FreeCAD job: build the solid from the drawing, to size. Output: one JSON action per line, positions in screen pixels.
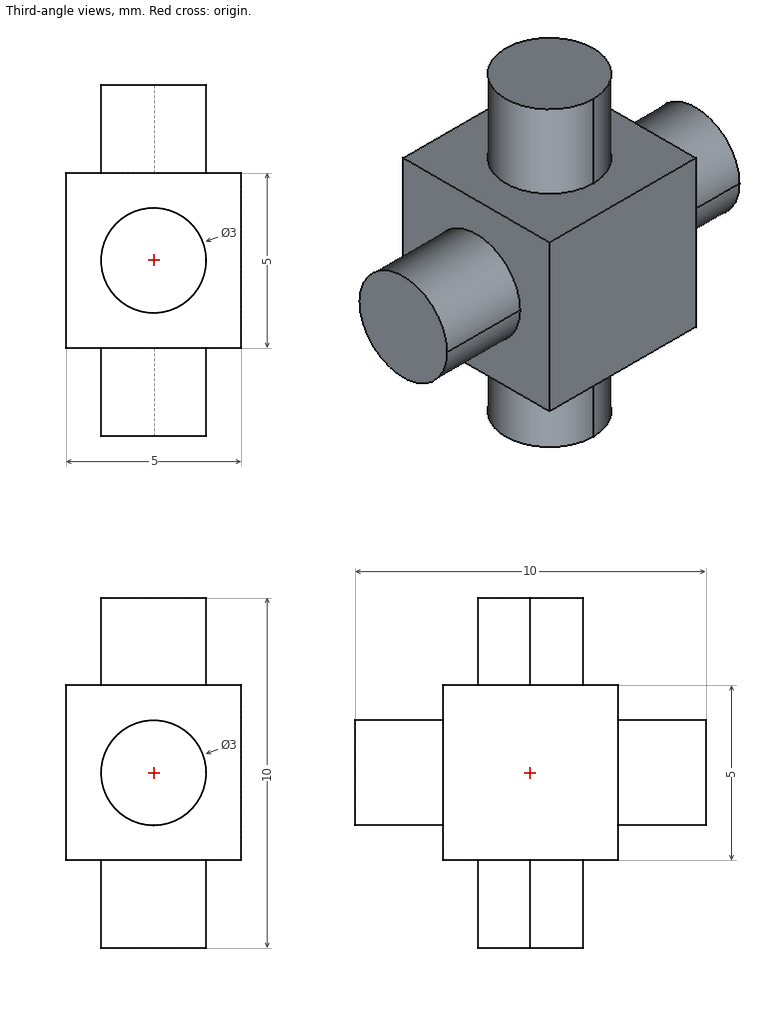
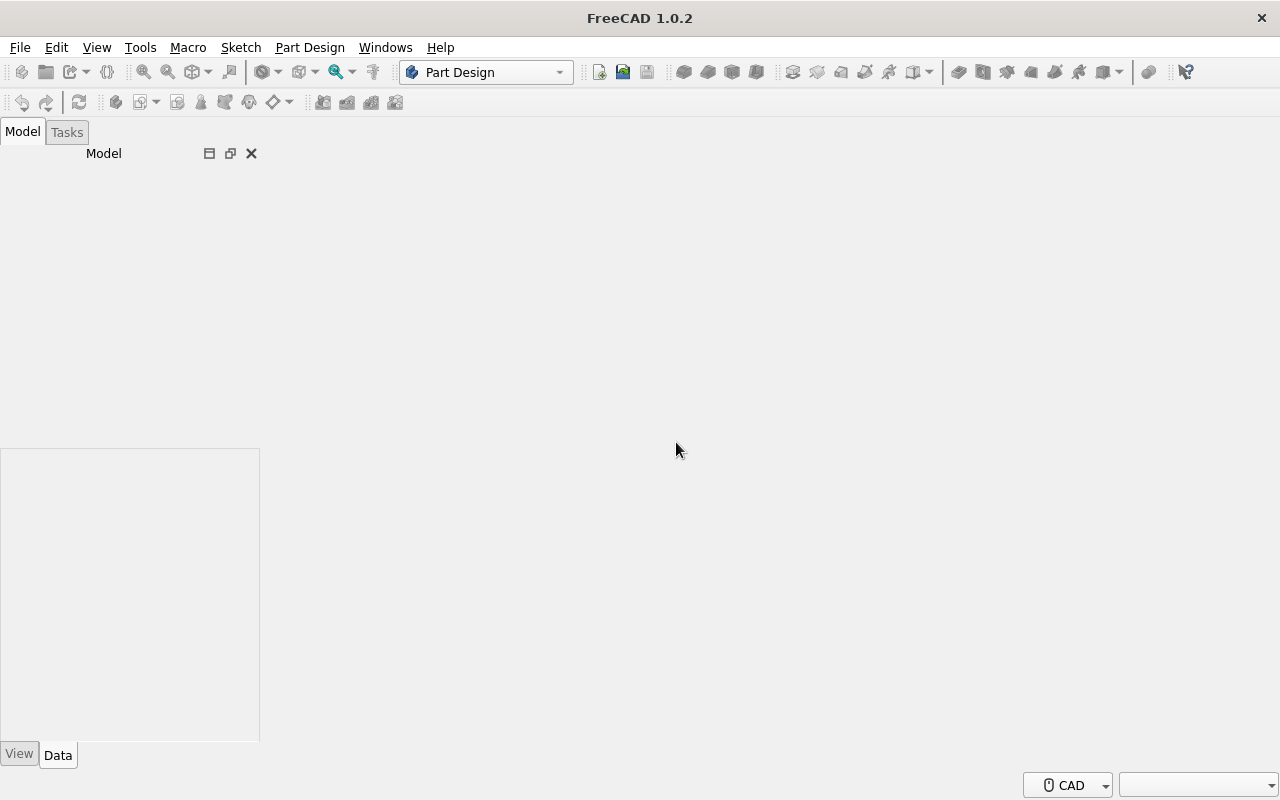
{"action": "left_click", "coordinate": [600, 72]}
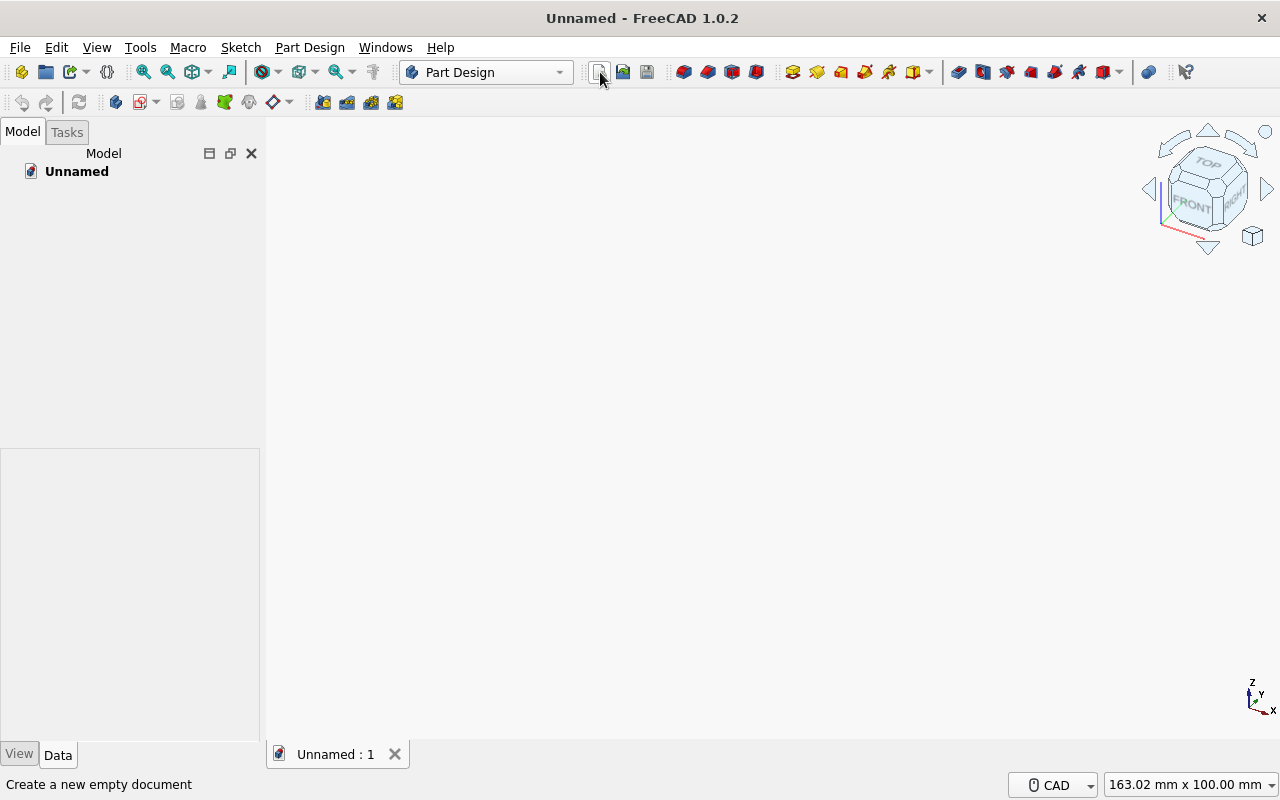
{"action": "left_click", "coordinate": [140, 102]}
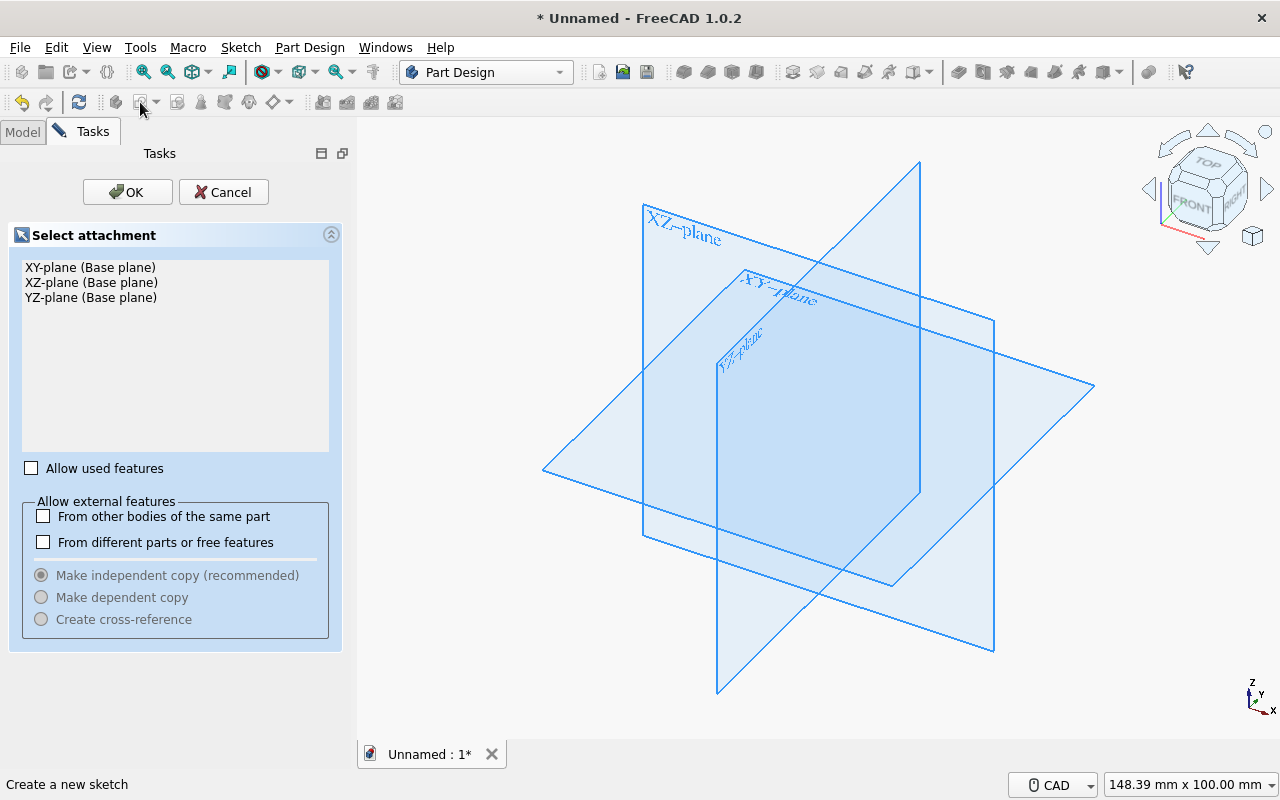
{"action": "left_click", "coordinate": [82, 268]}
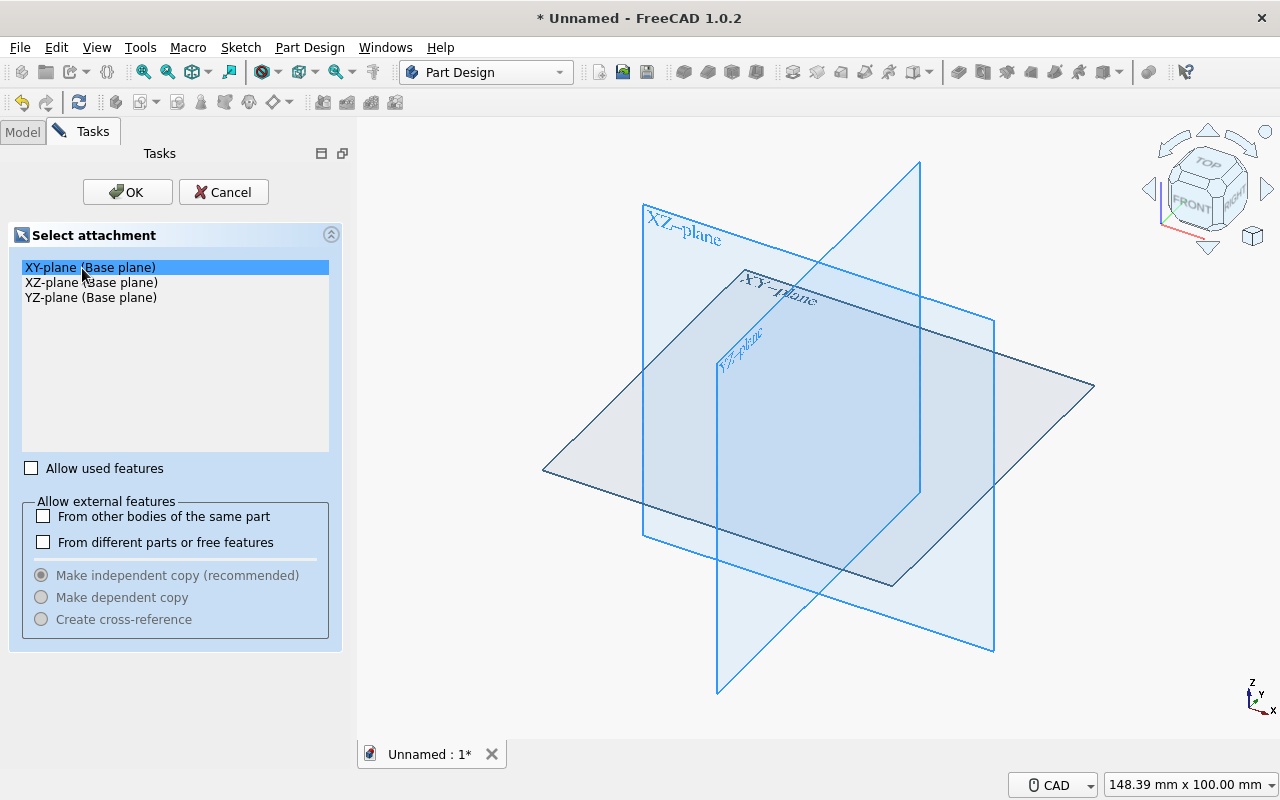
{"action": "left_click", "coordinate": [128, 192]}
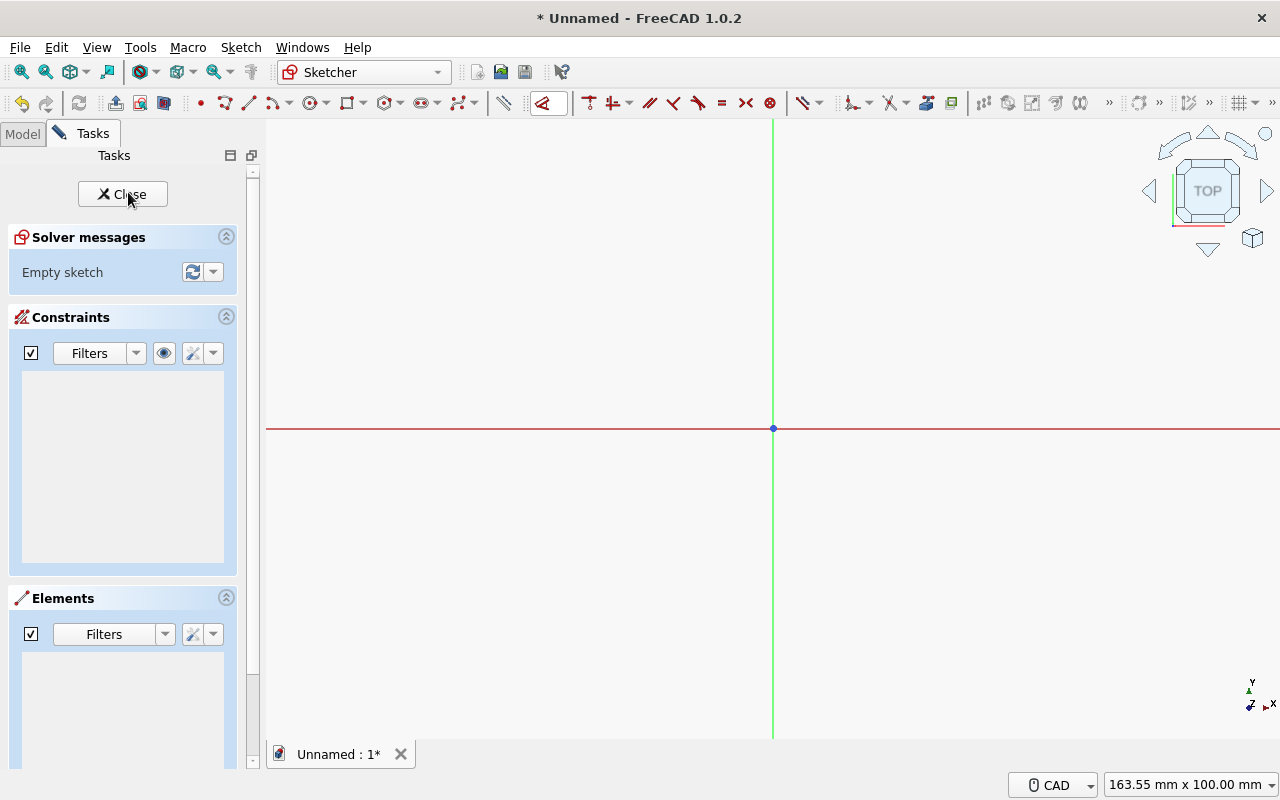
{"action": "scroll", "coordinate": [778, 429], "scroll_direction": "up", "scroll_amount": 13}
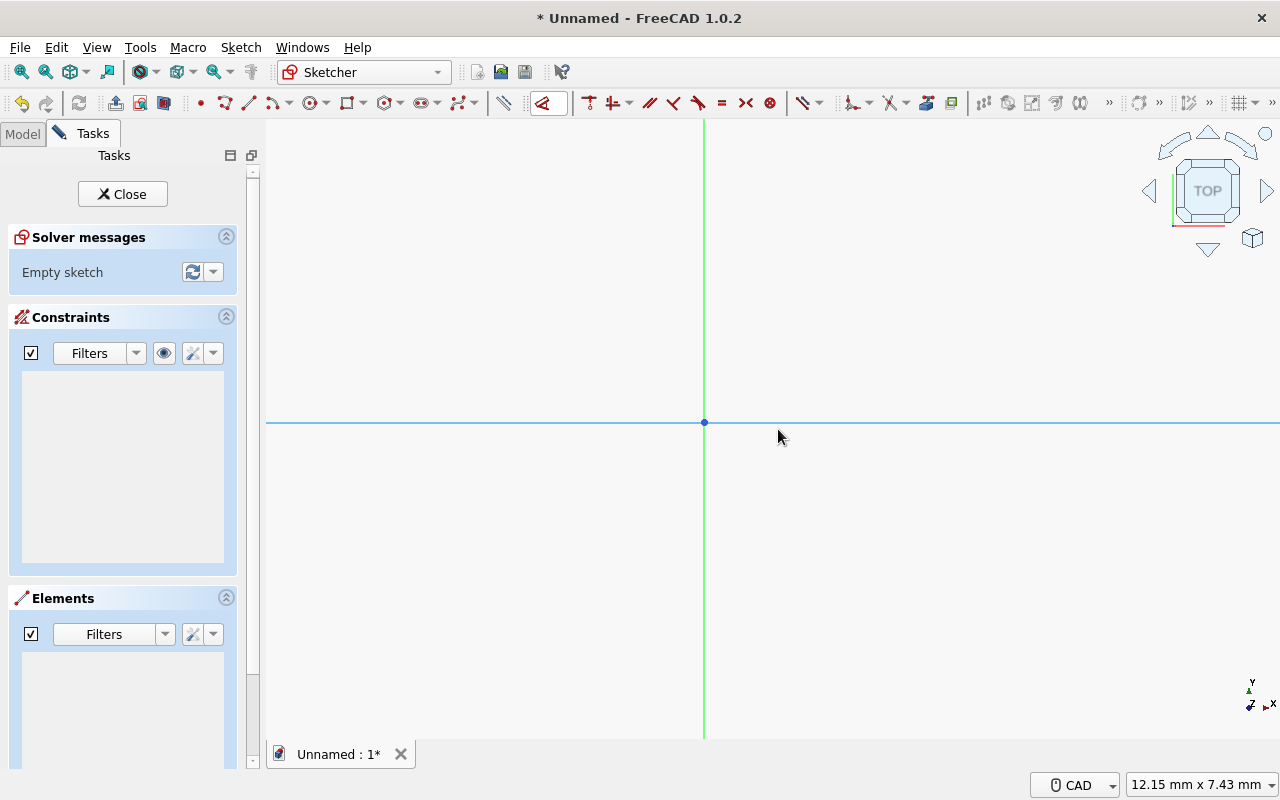
{"action": "key", "text": "g v"}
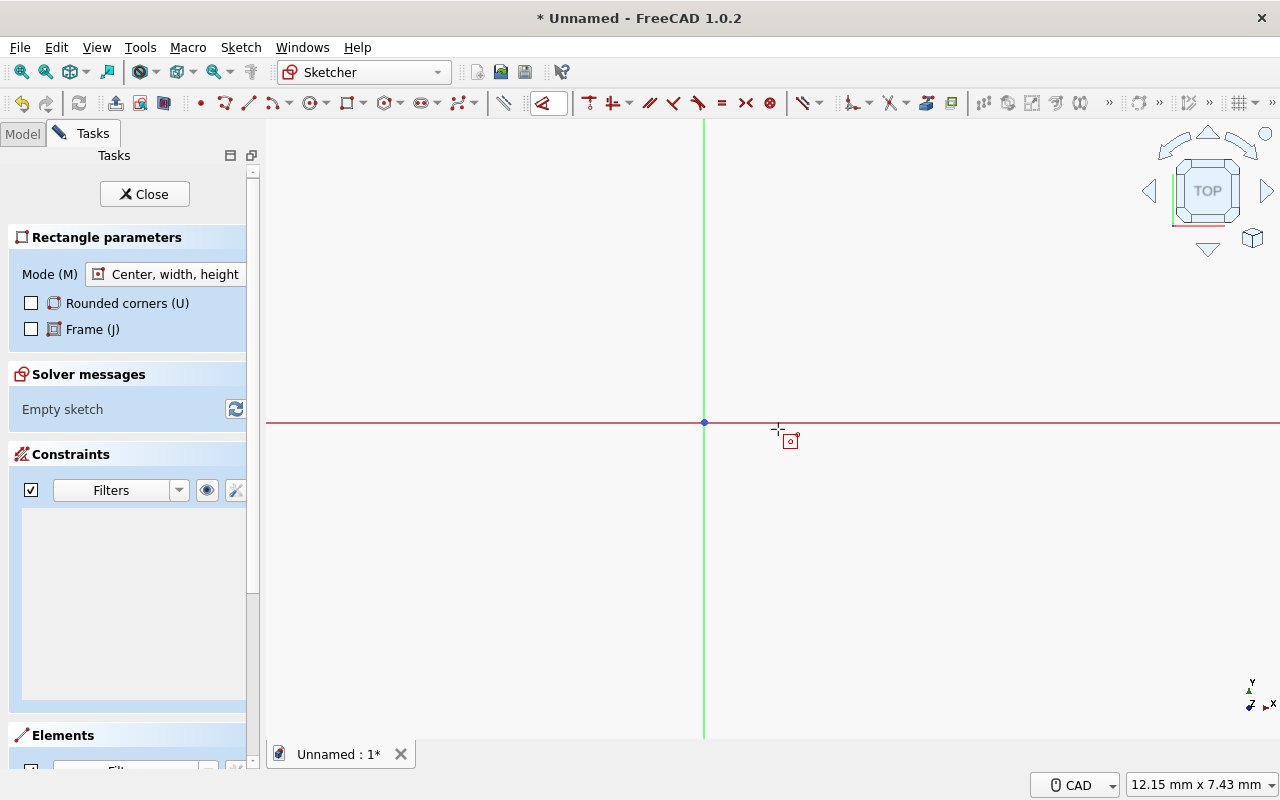
{"action": "left_click", "coordinate": [704, 423]}
{"action": "mouse_move", "coordinate": [913, 214]}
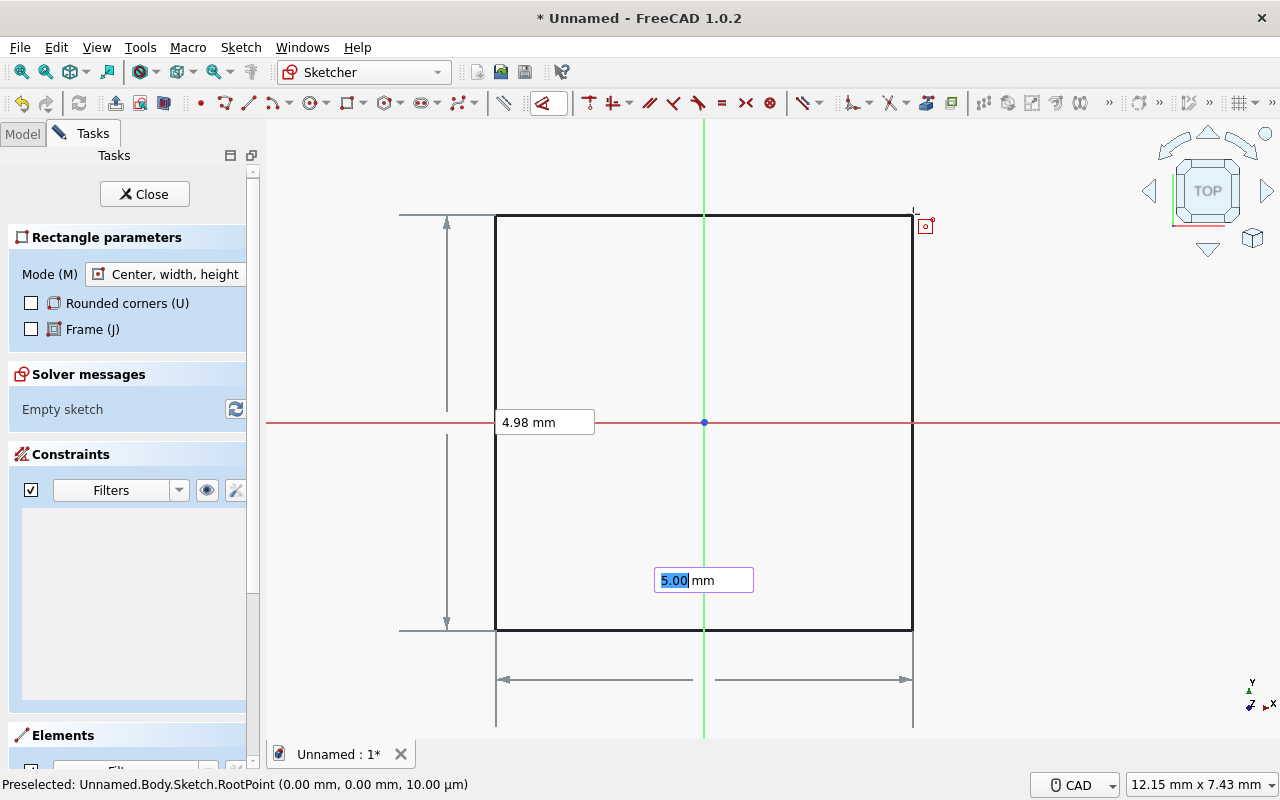
{"action": "type", "text": "5"}
{"action": "key", "text": "Tab"}
{"action": "type", "text": "5"}
{"action": "key", "text": "Return"}
{"action": "key", "text": "Escape"}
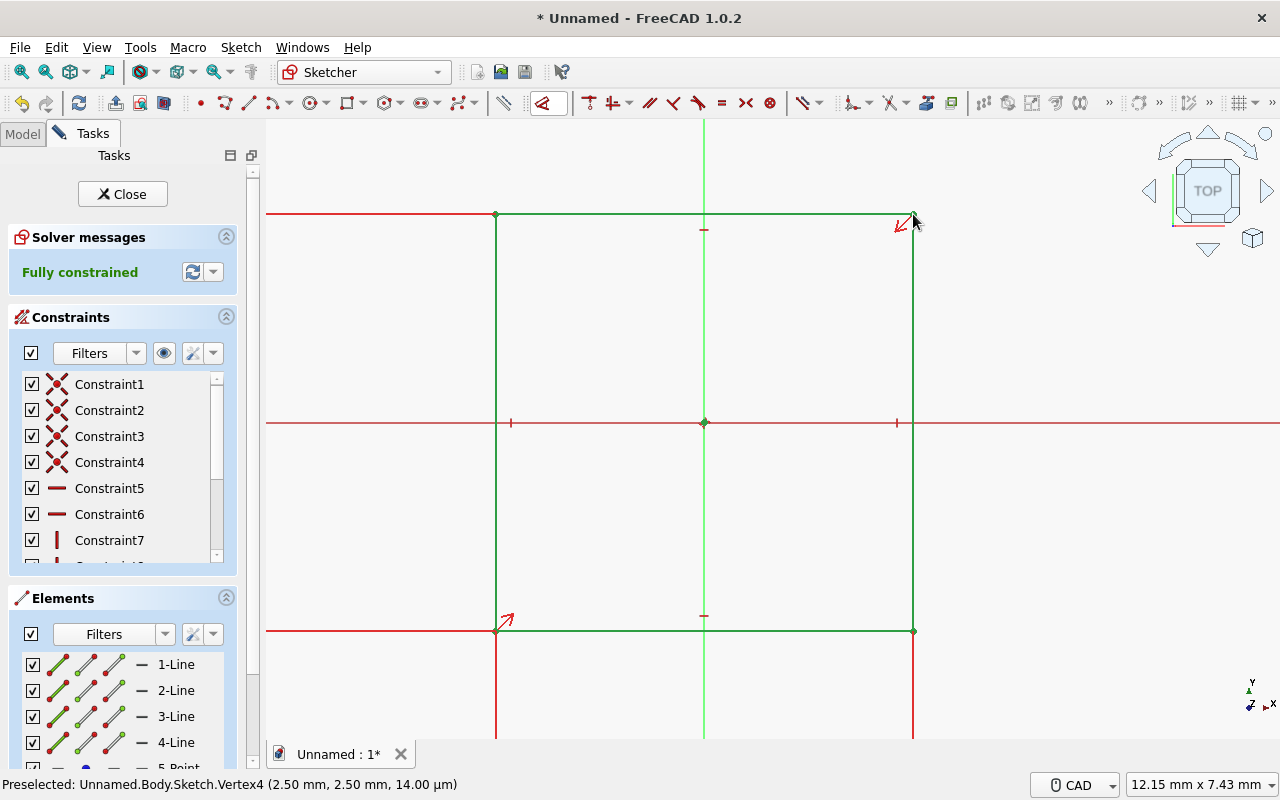
{"action": "left_click", "coordinate": [123, 194]}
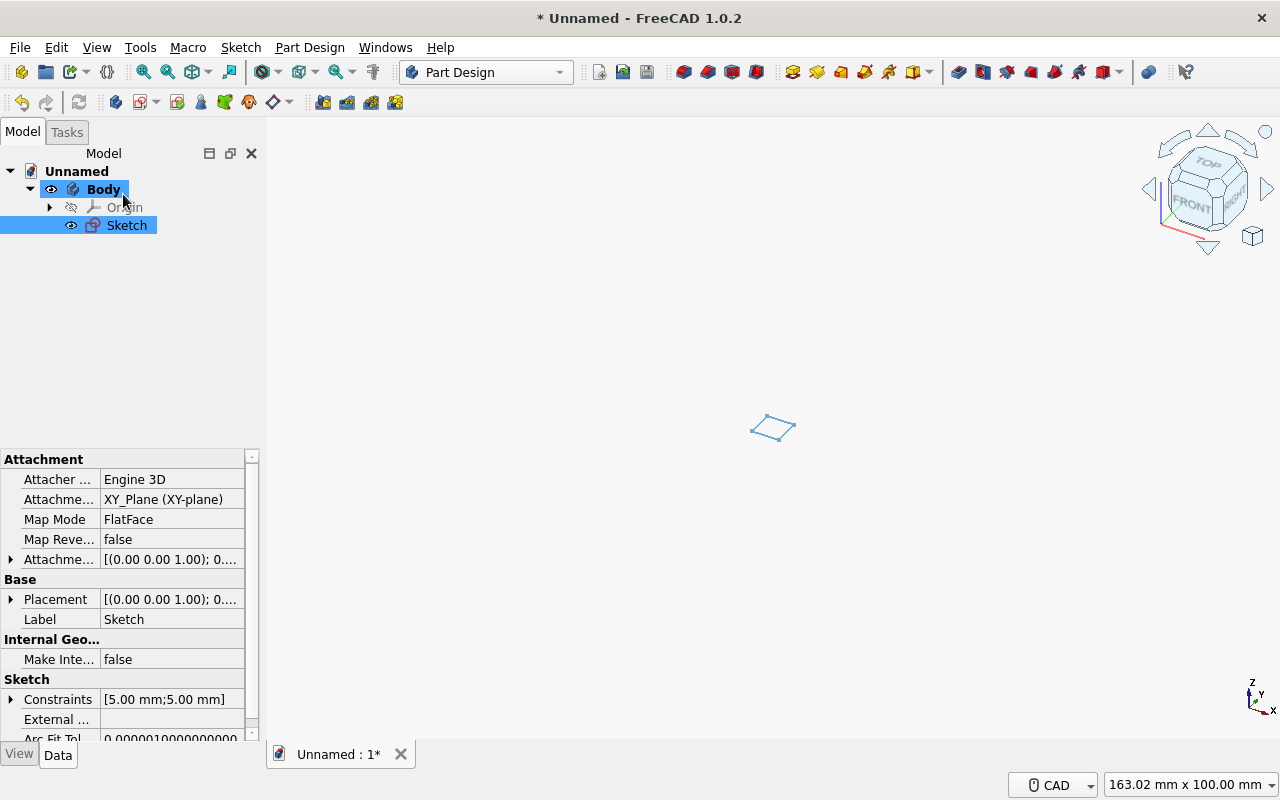
{"action": "left_click", "coordinate": [794, 72]}